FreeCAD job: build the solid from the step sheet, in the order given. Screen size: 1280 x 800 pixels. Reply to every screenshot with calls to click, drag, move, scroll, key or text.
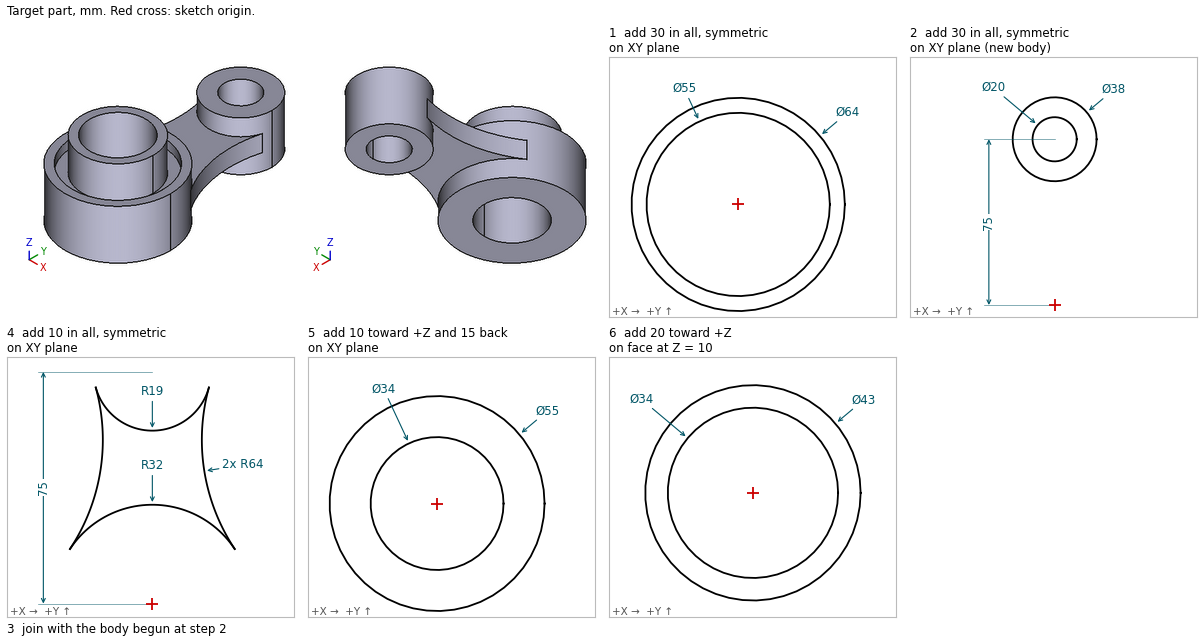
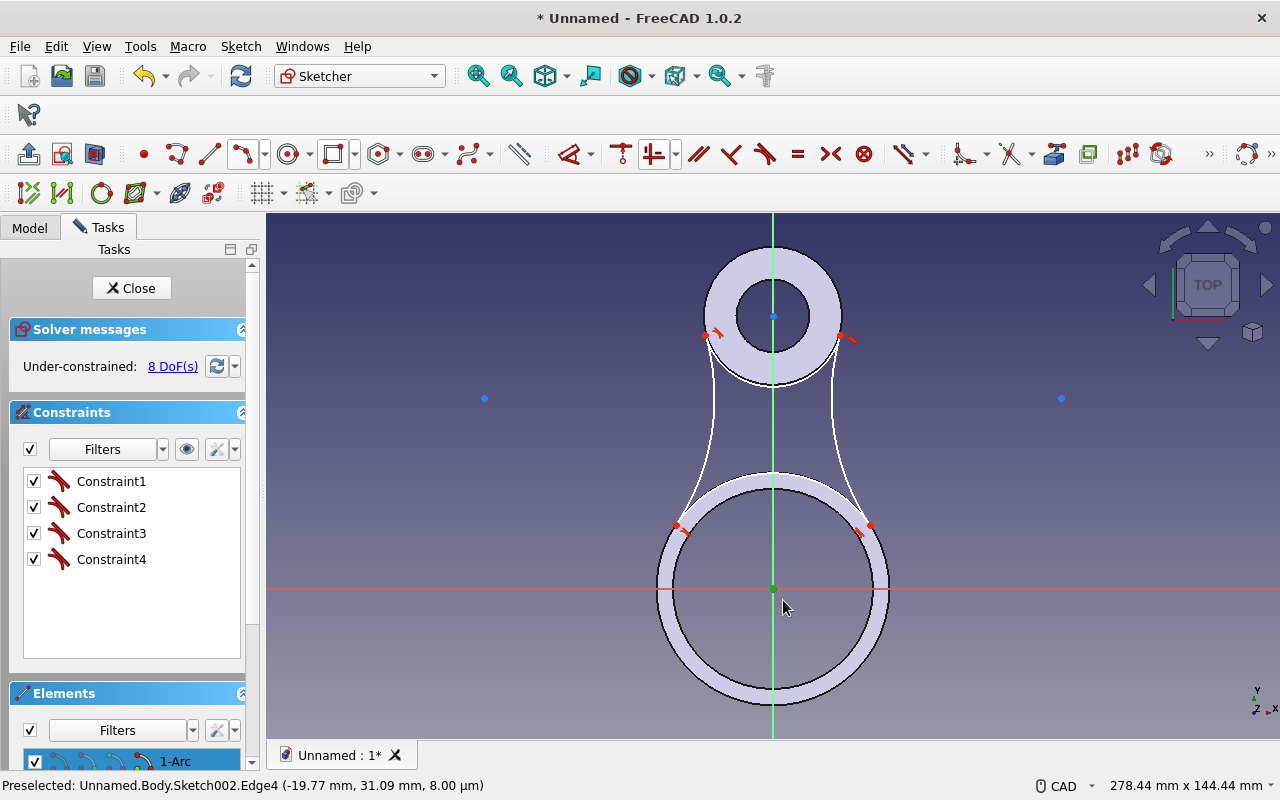
key(c)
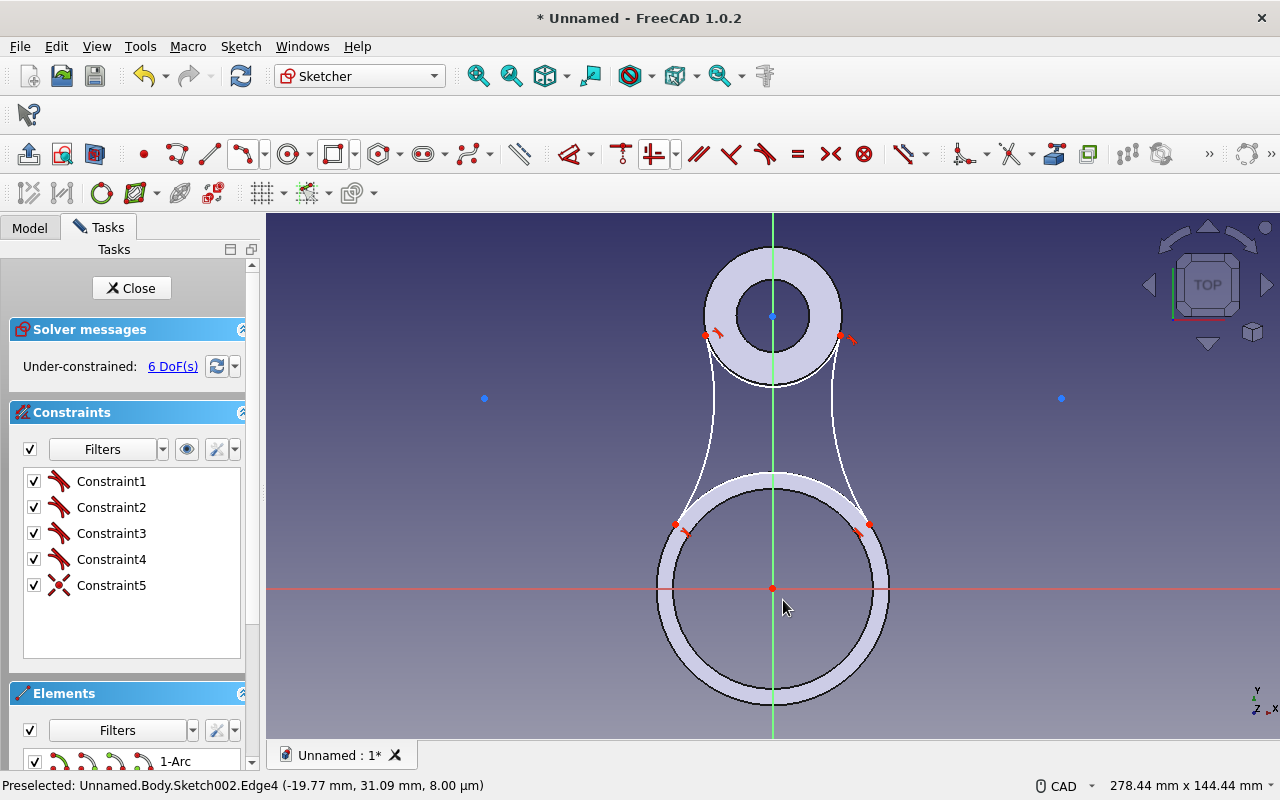
click(832, 394)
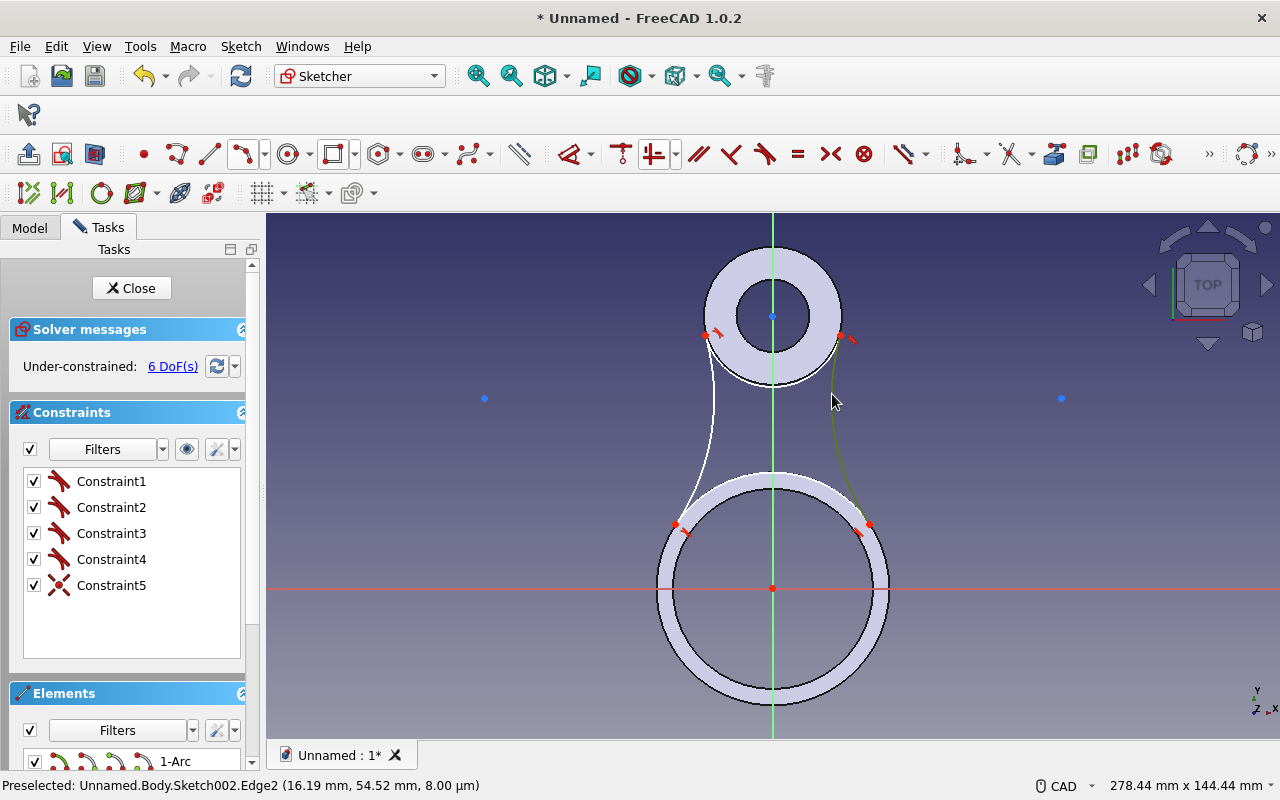
click(702, 472)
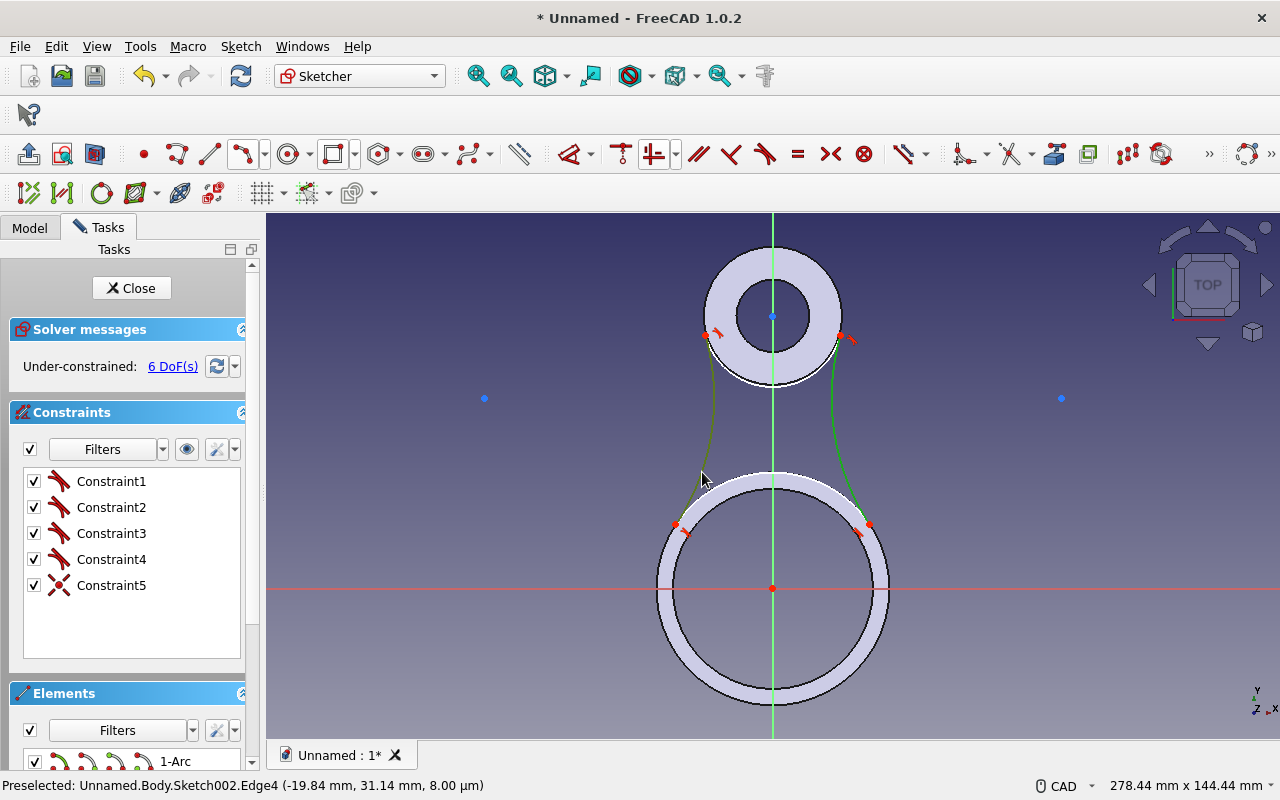
click(798, 154)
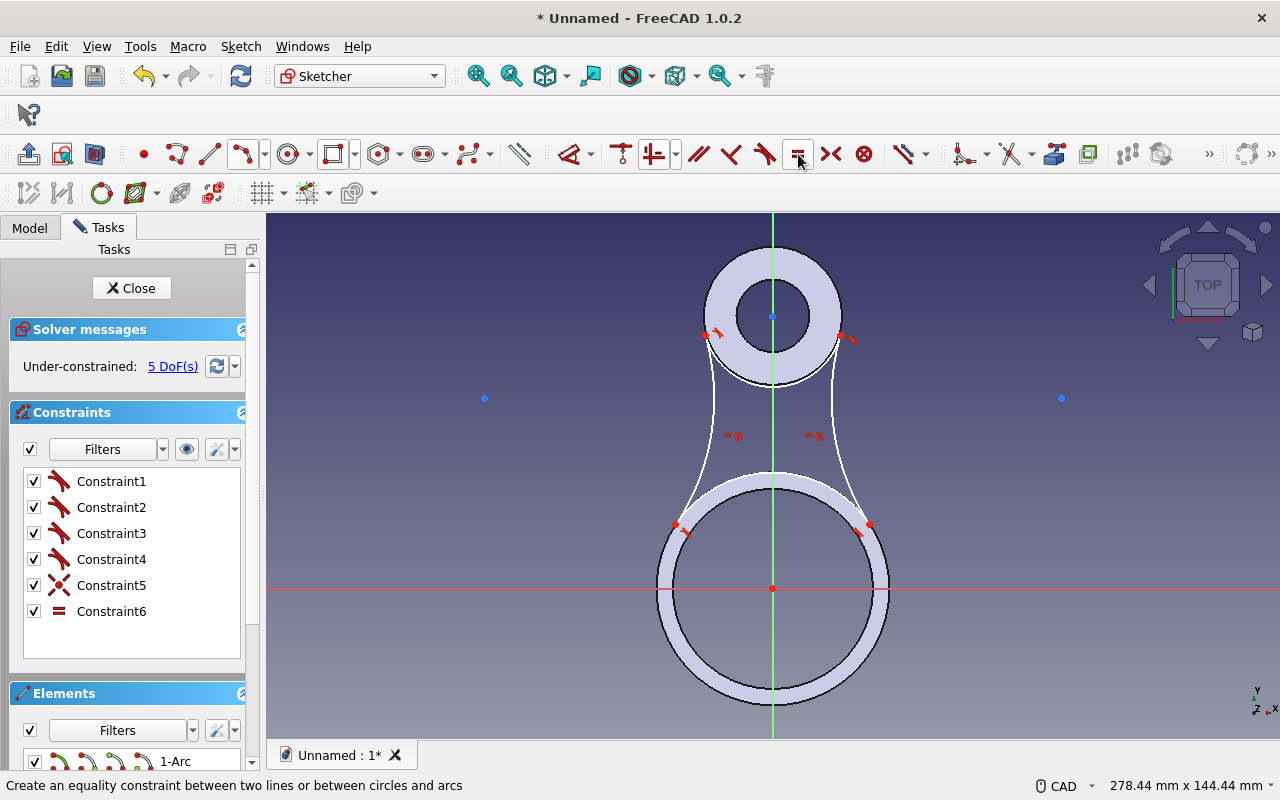
click(773, 317)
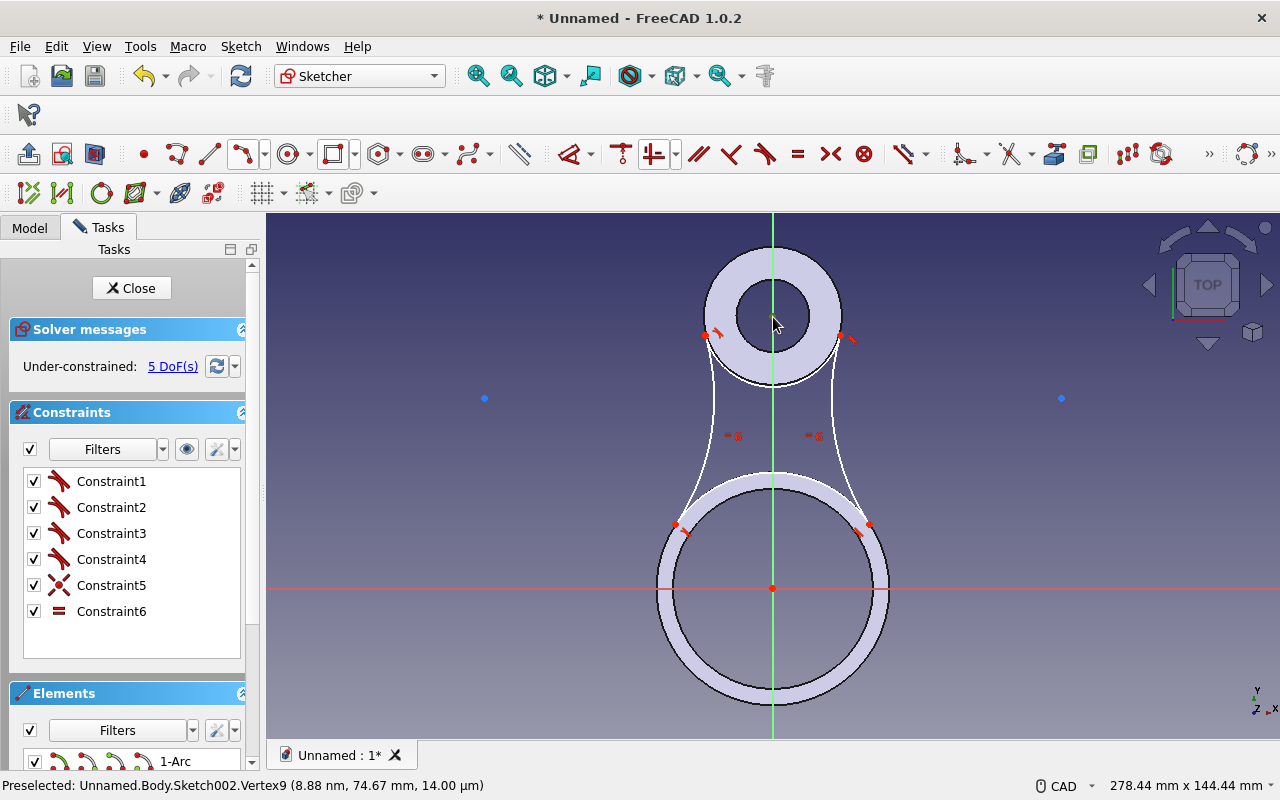
click(773, 677)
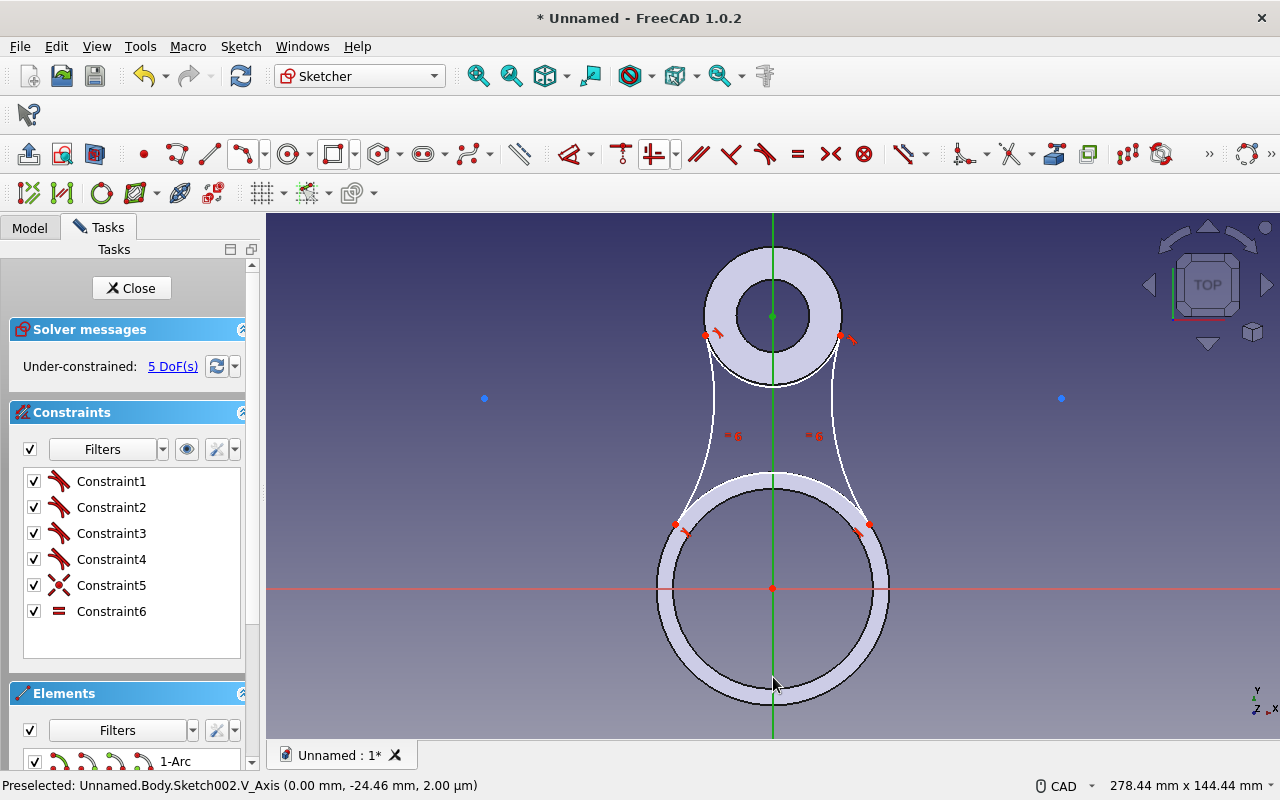
key(c)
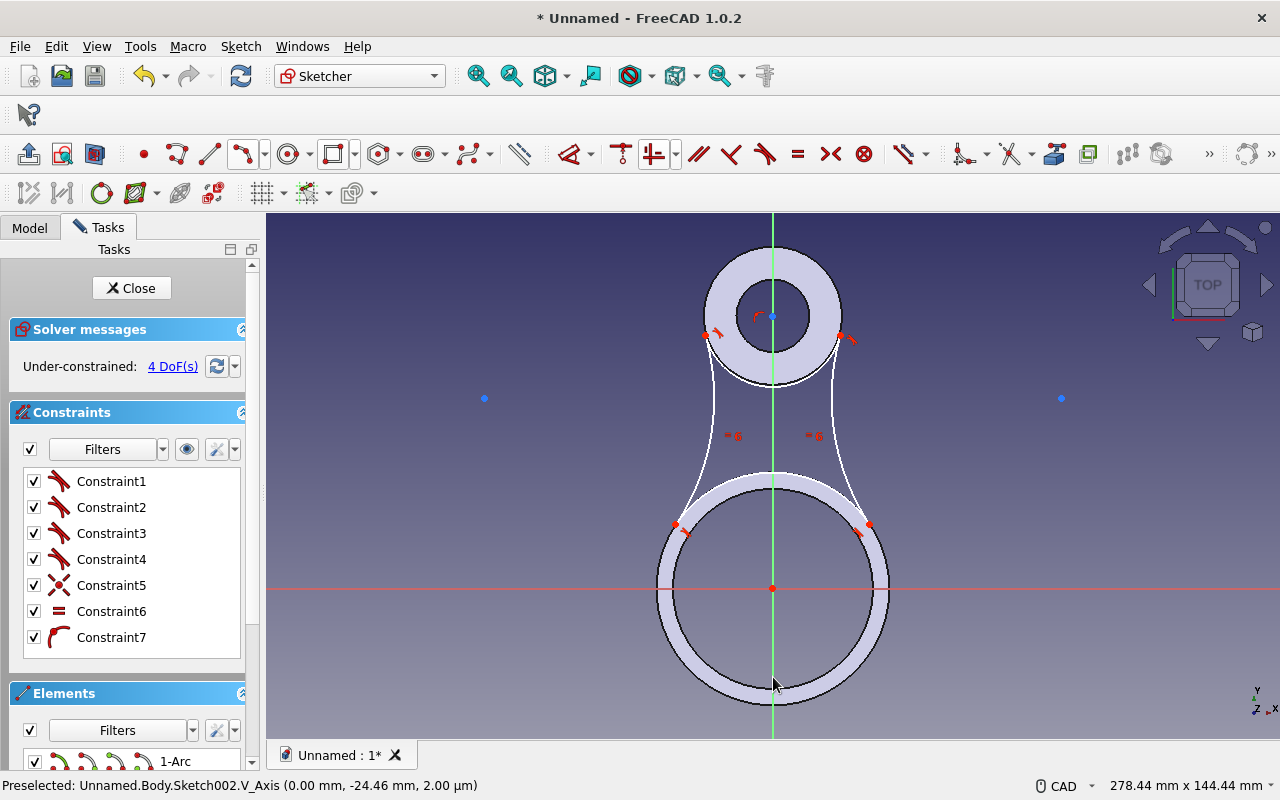
key(d)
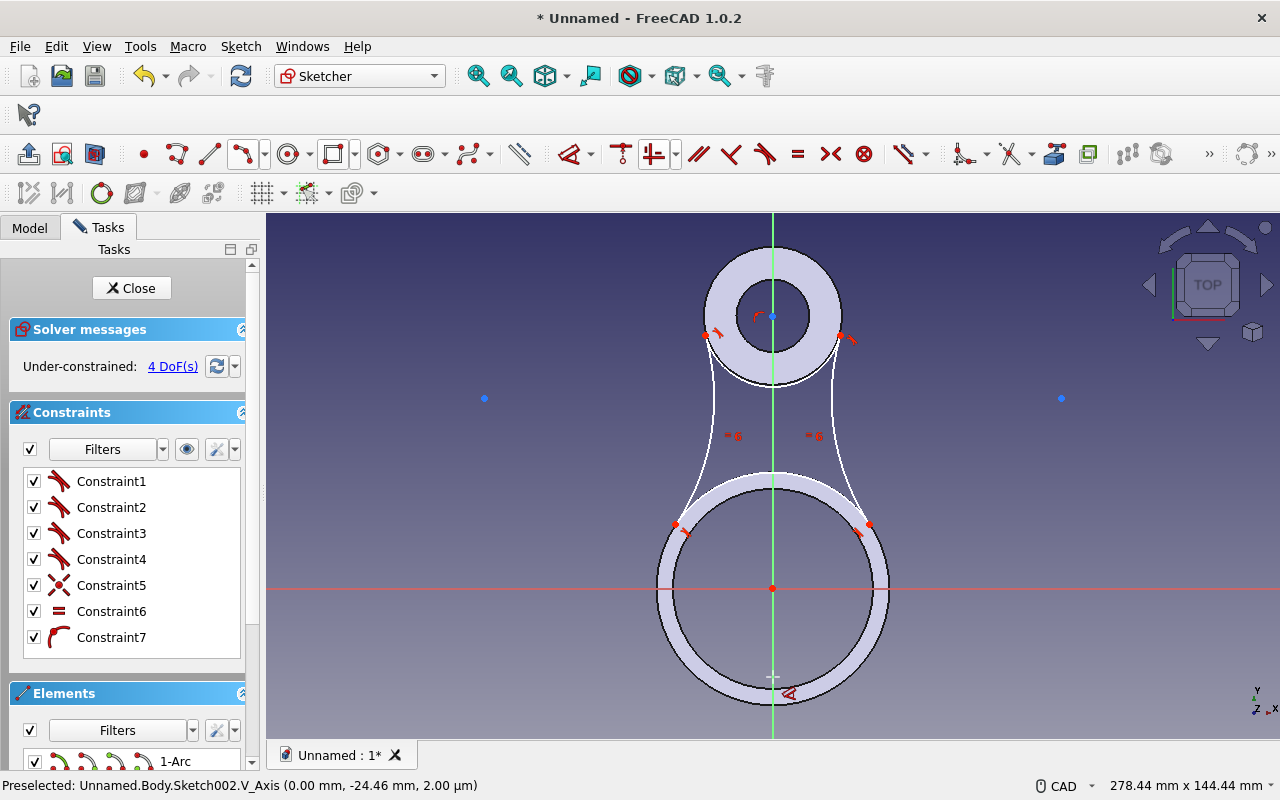
click(818, 482)
click(889, 497)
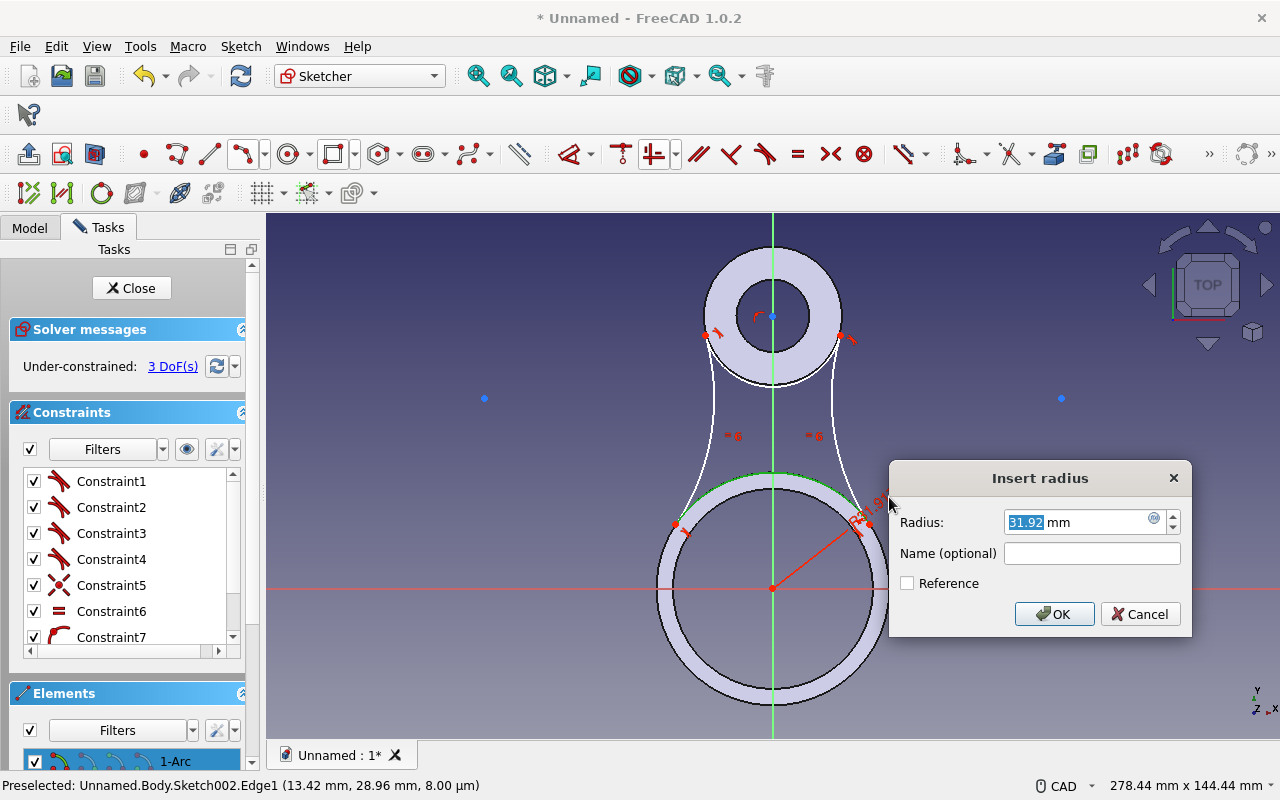
text(32)
key(Return)